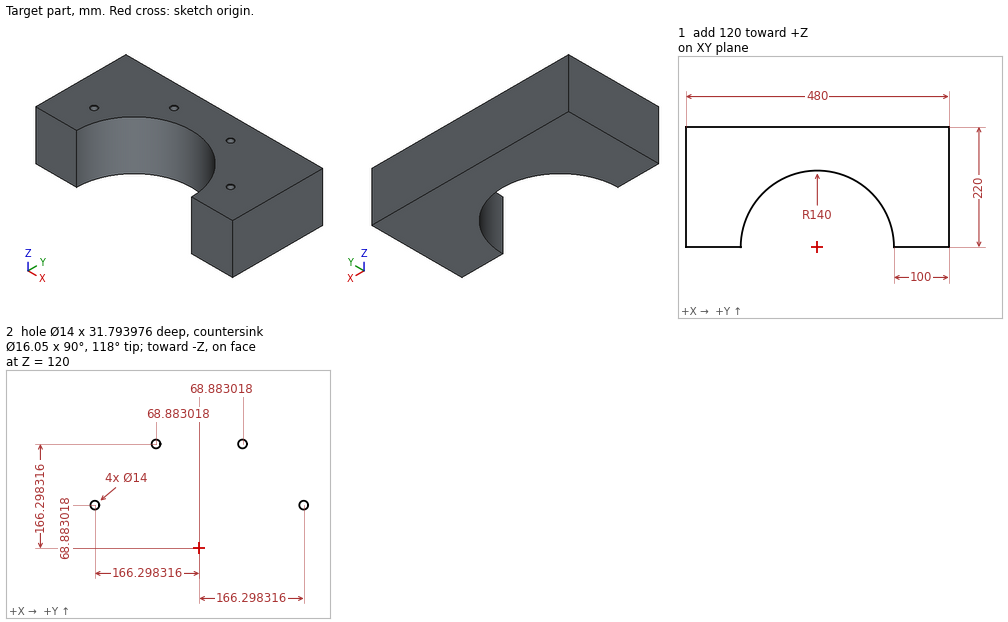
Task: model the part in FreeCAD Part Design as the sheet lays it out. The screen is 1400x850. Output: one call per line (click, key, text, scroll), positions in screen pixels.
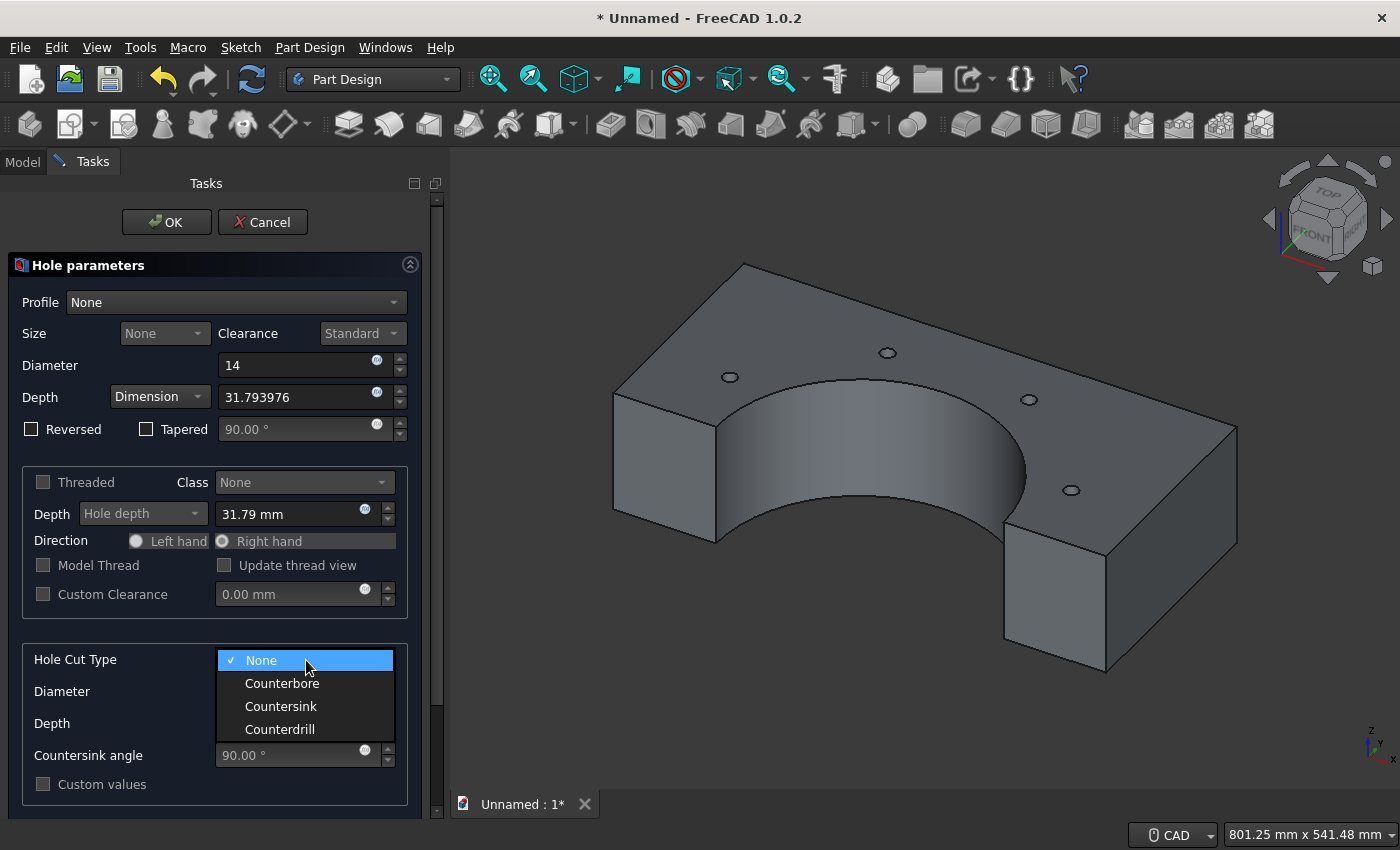
click(304, 706)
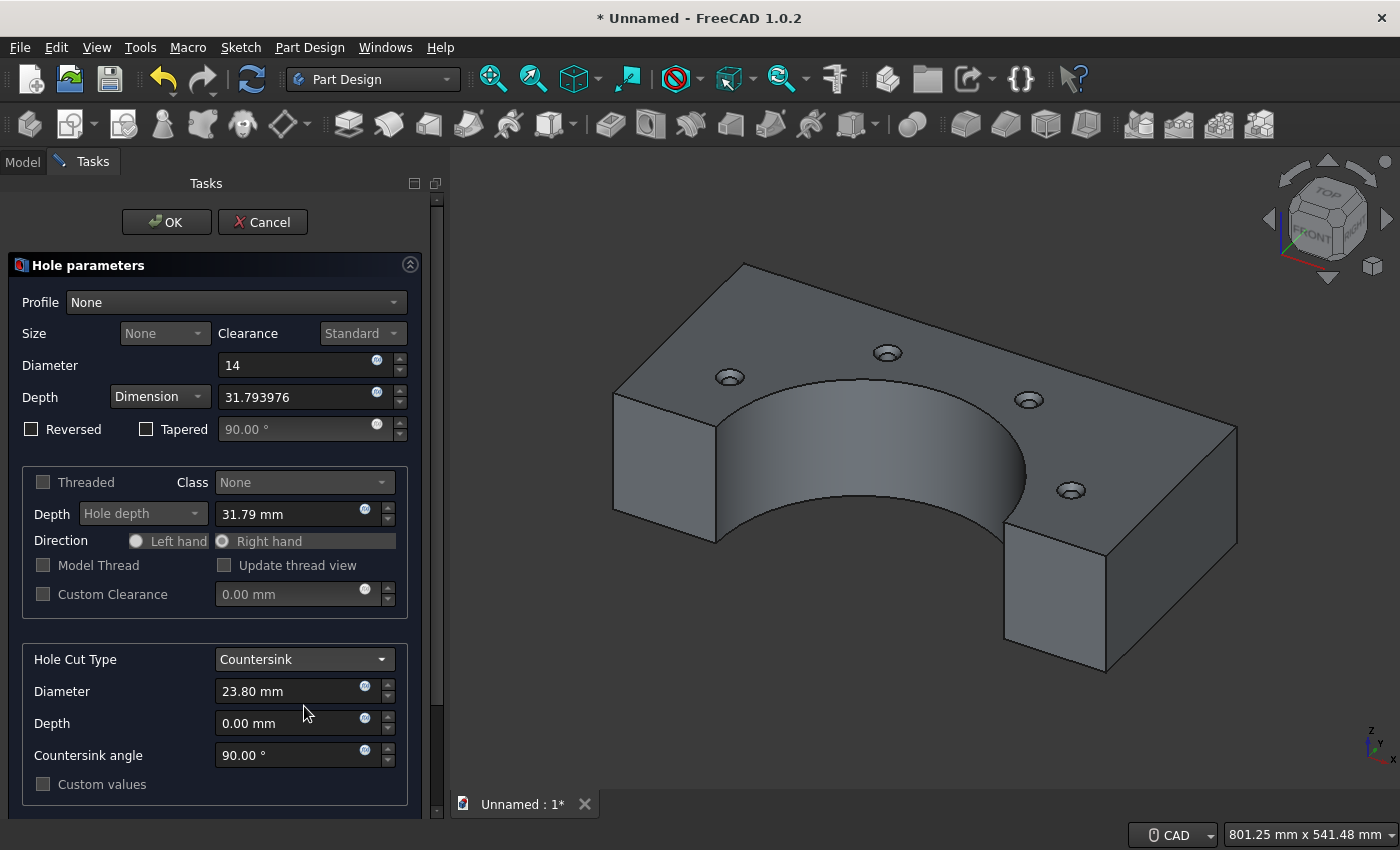
triple_click(298, 691)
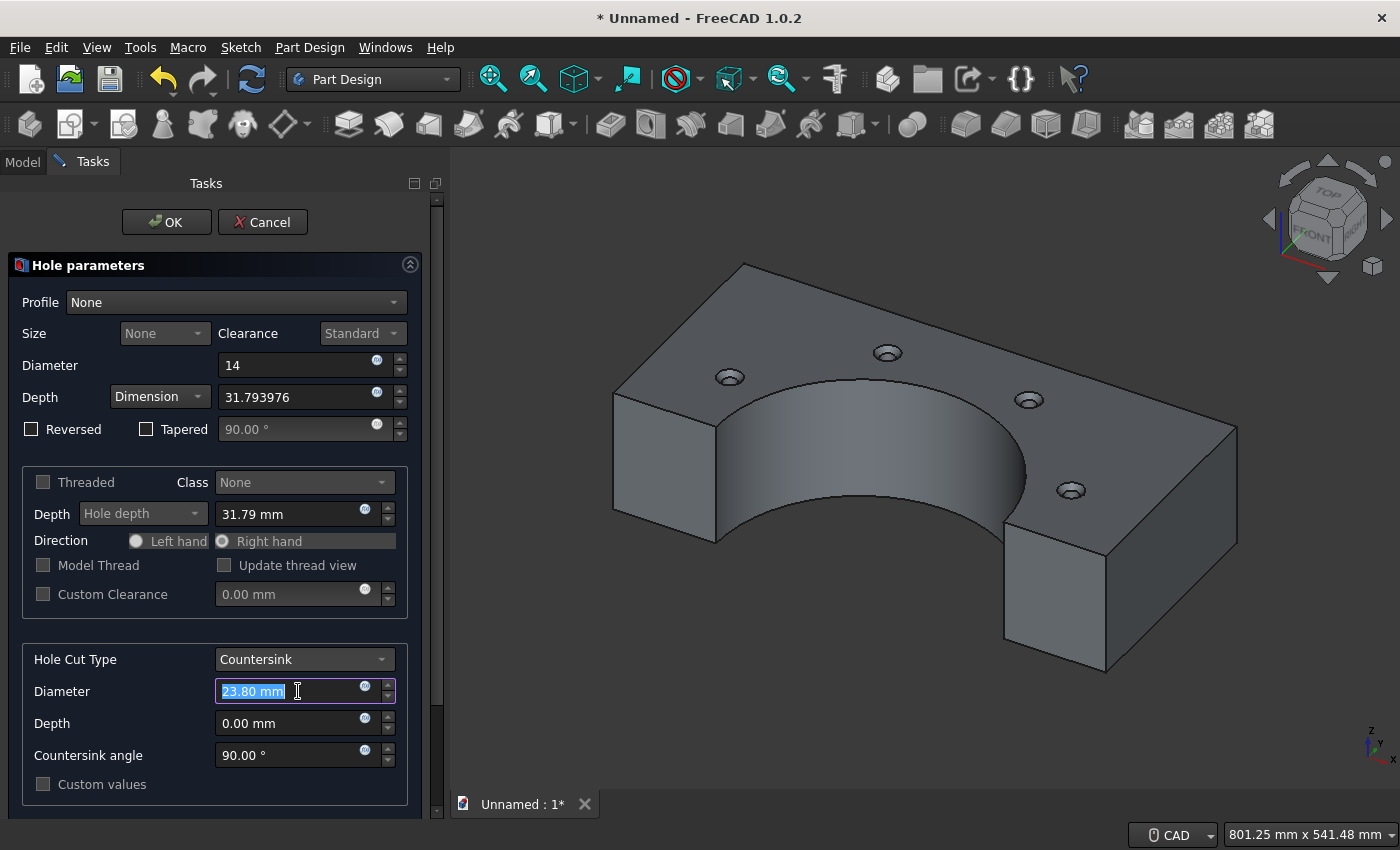
text(16.05)
key(Tab)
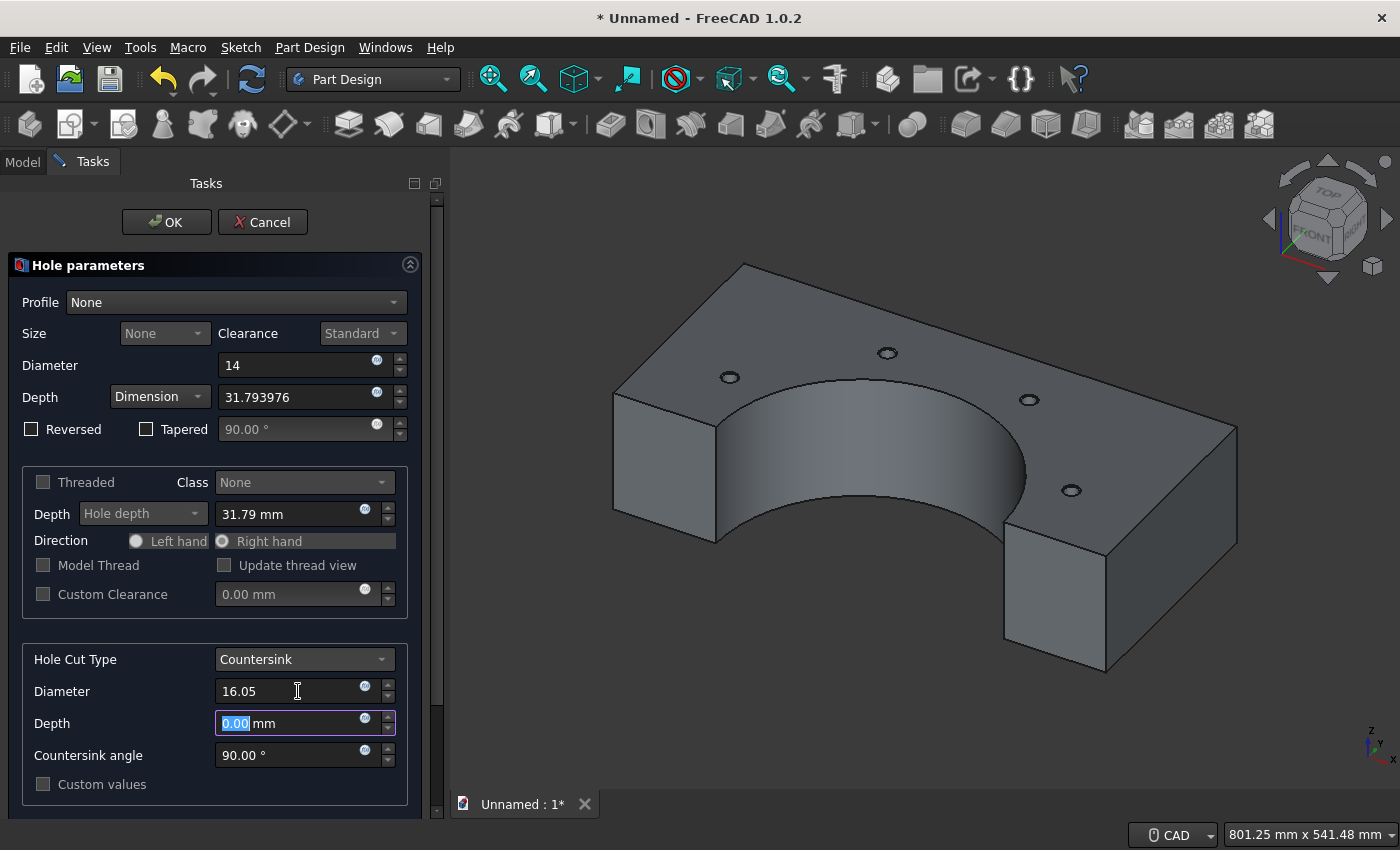
click(167, 222)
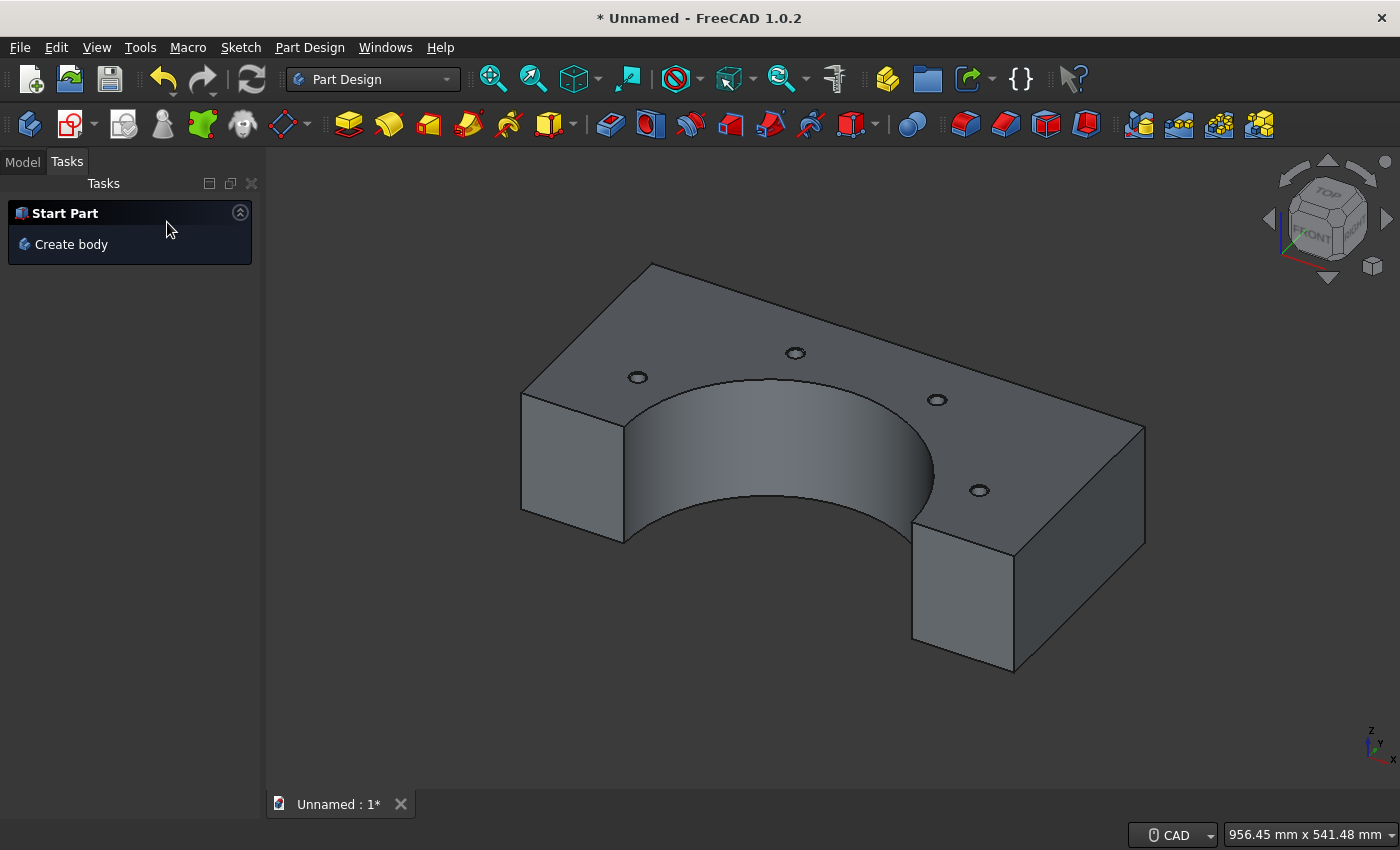
key(0)